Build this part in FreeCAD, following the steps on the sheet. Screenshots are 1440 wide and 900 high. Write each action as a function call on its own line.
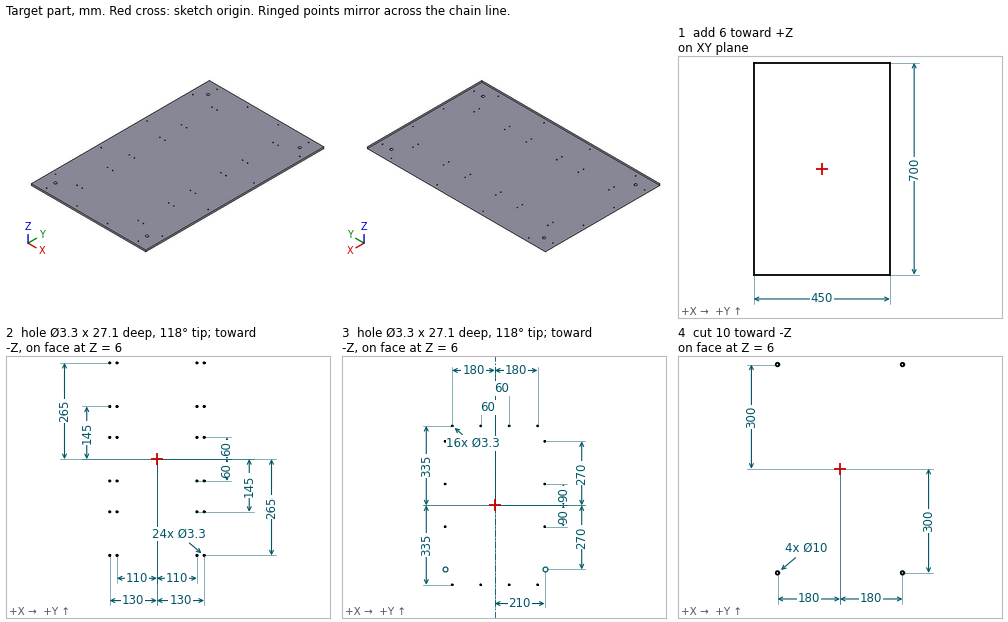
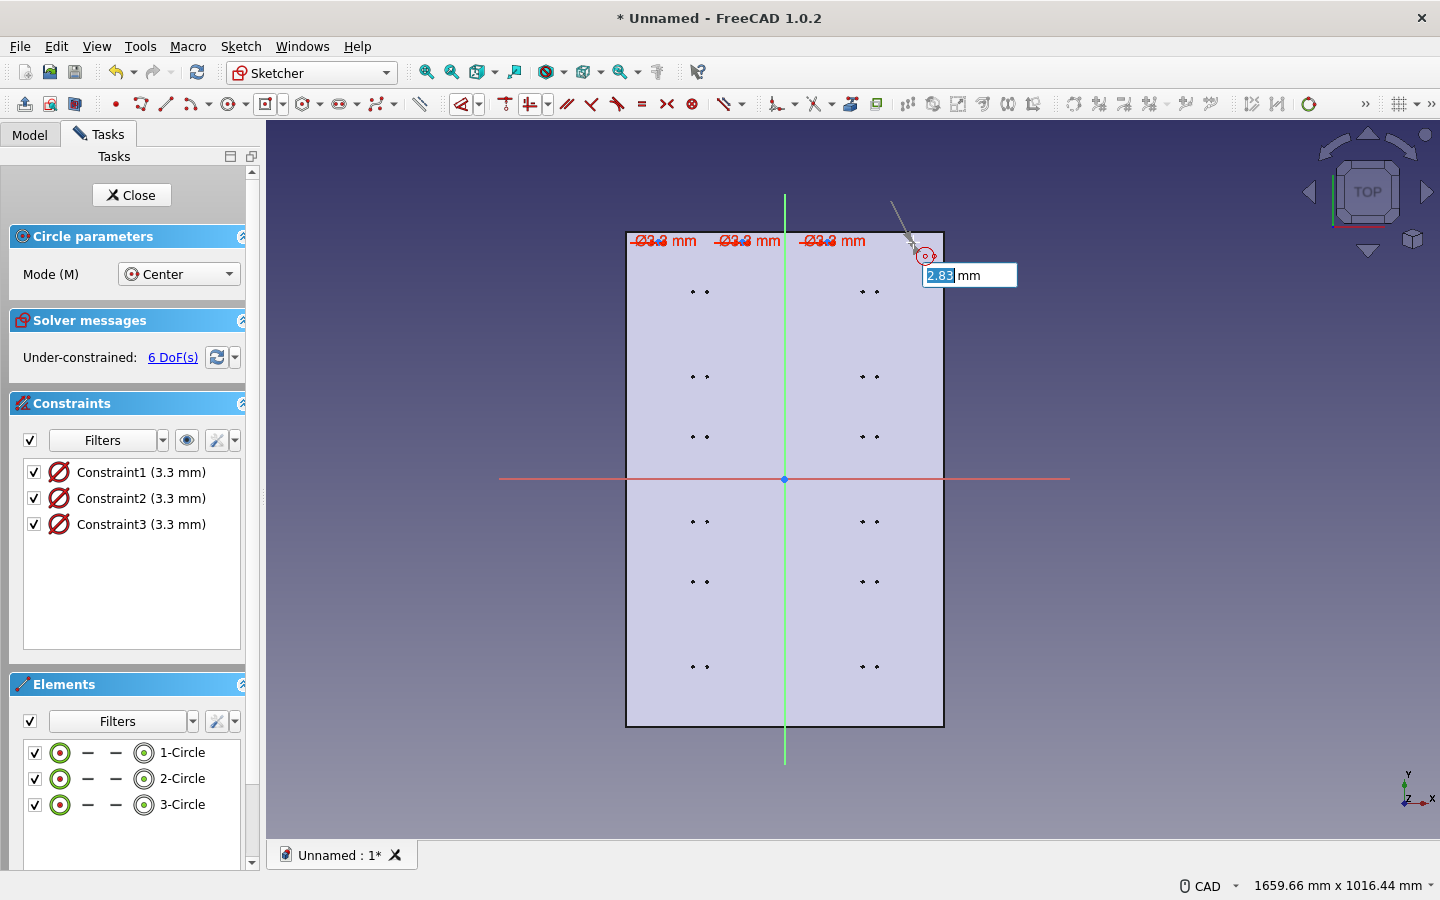
text(3.3)
key(Return)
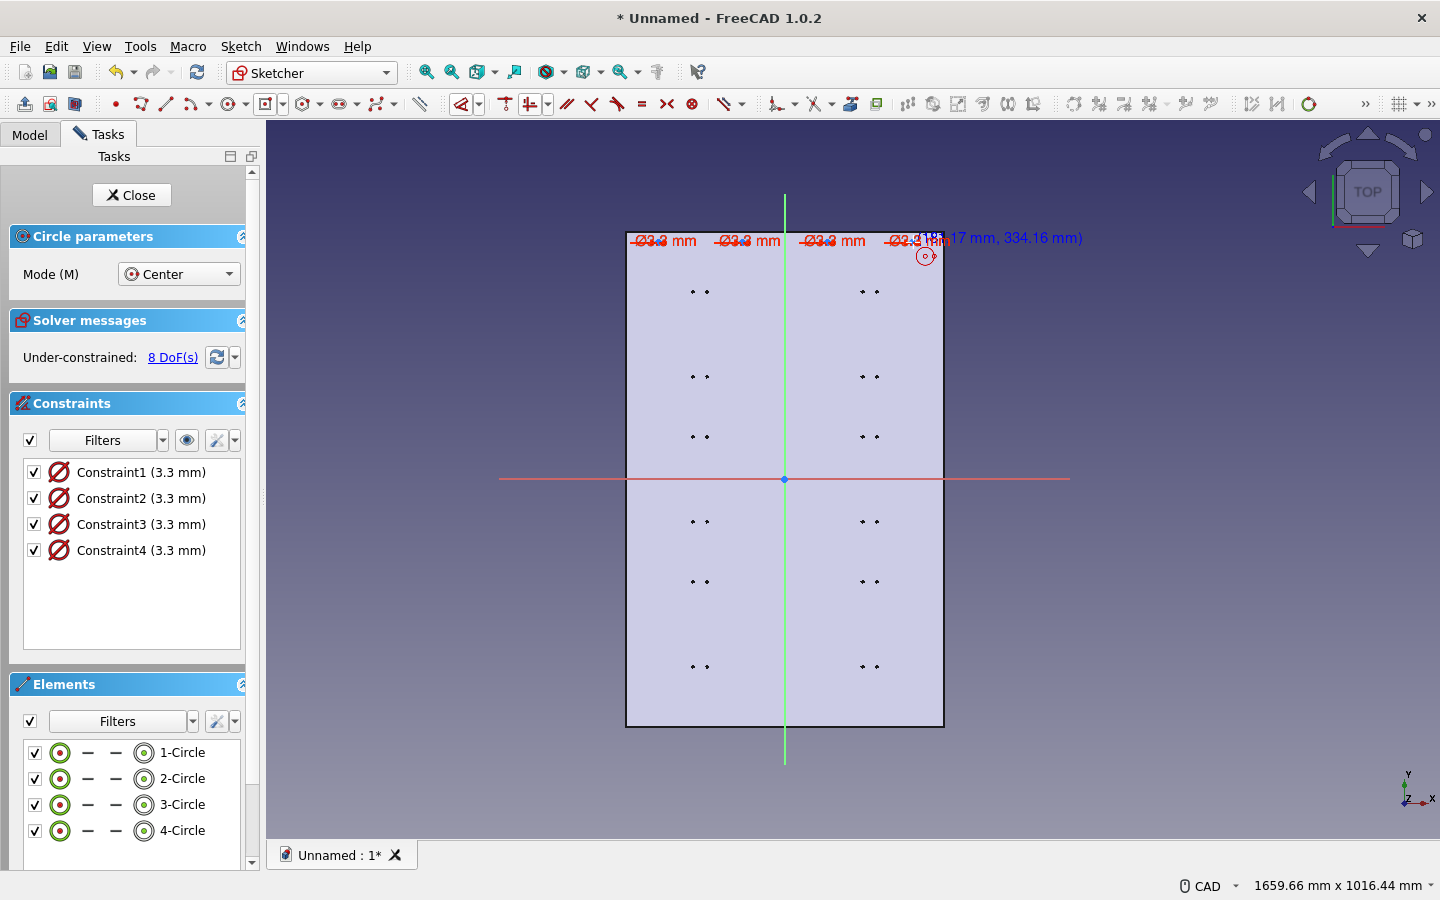
scroll(658, 716, up, 15)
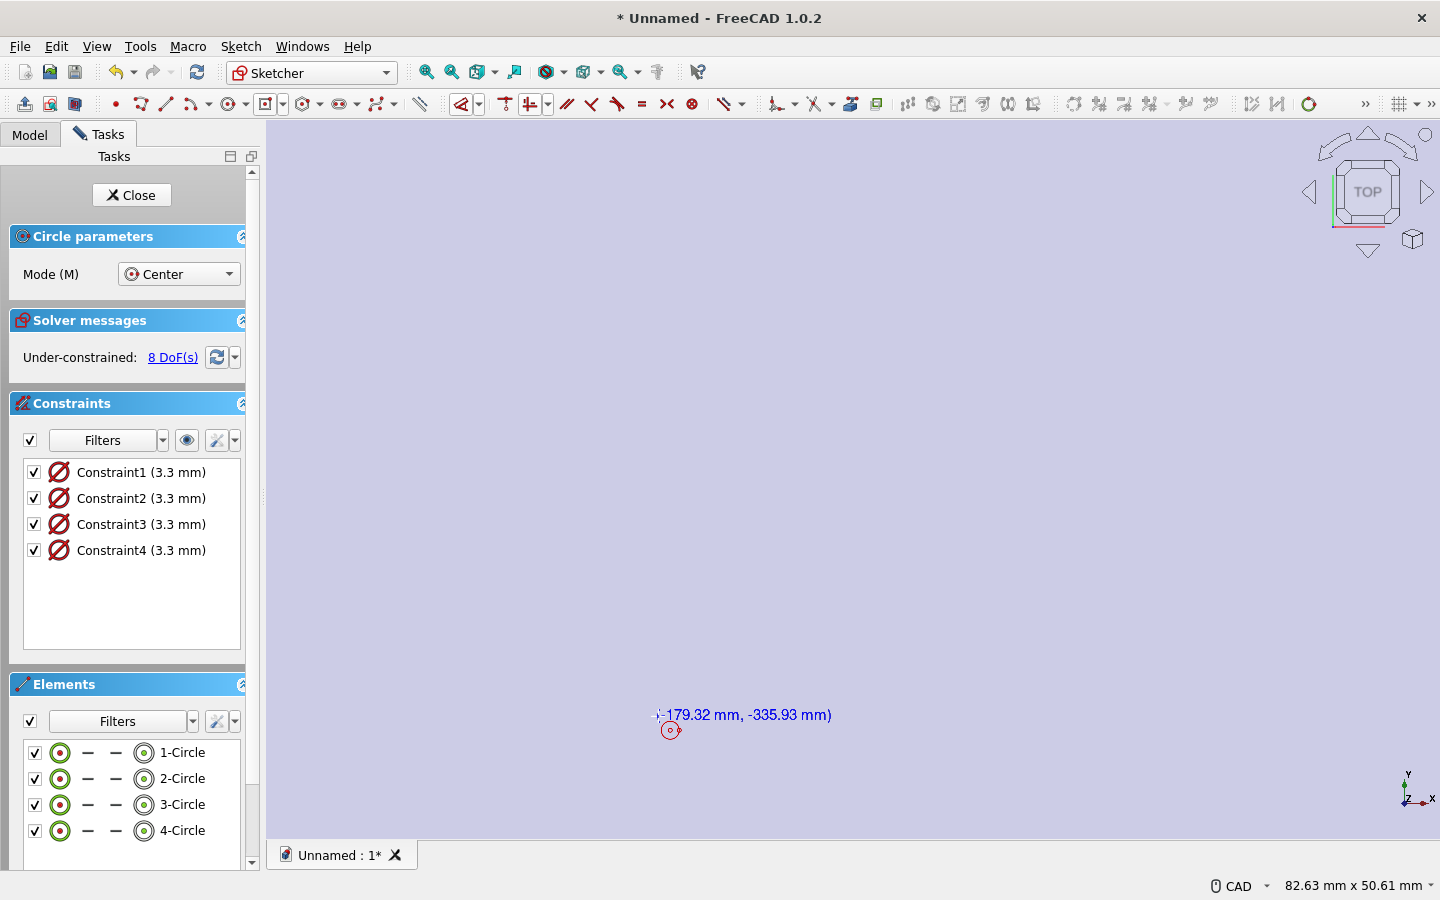
scroll(658, 717, down, 15)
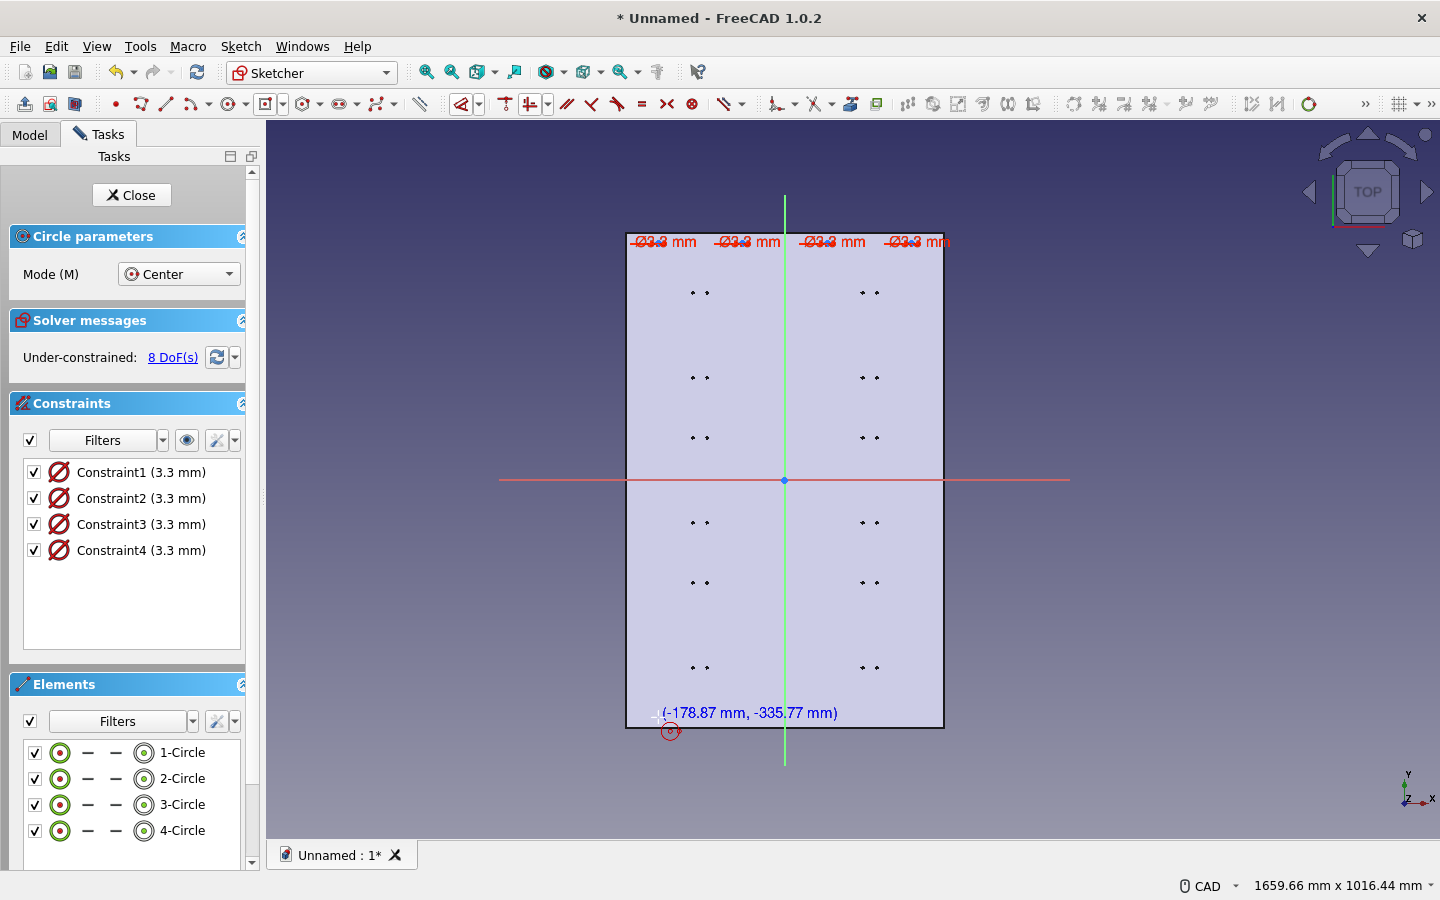
click(658, 717)
move(658, 716)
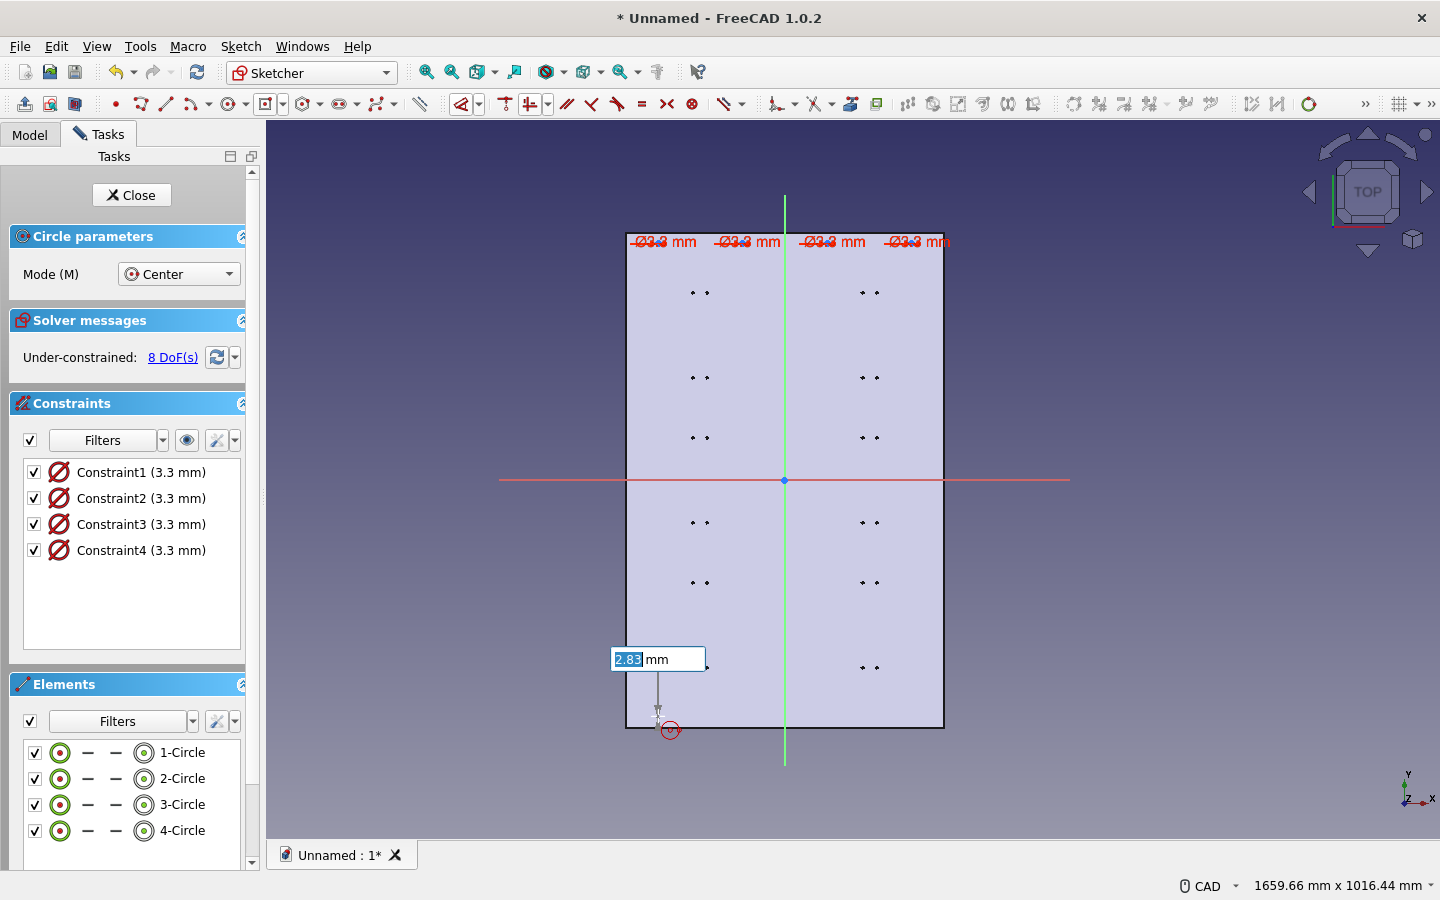
text(3.3)
key(Return)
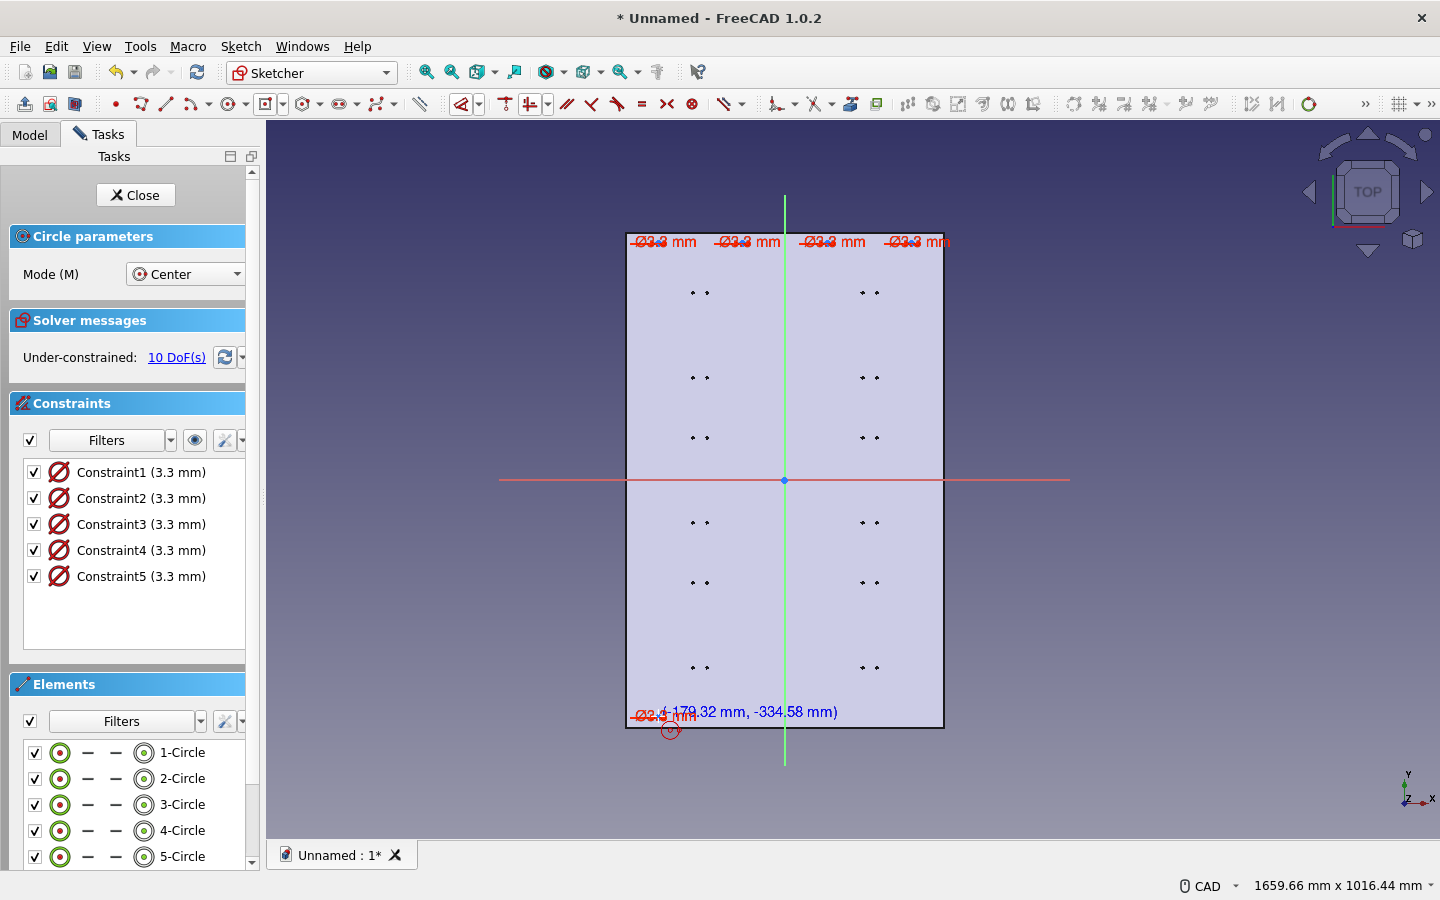
scroll(742, 717, up, 15)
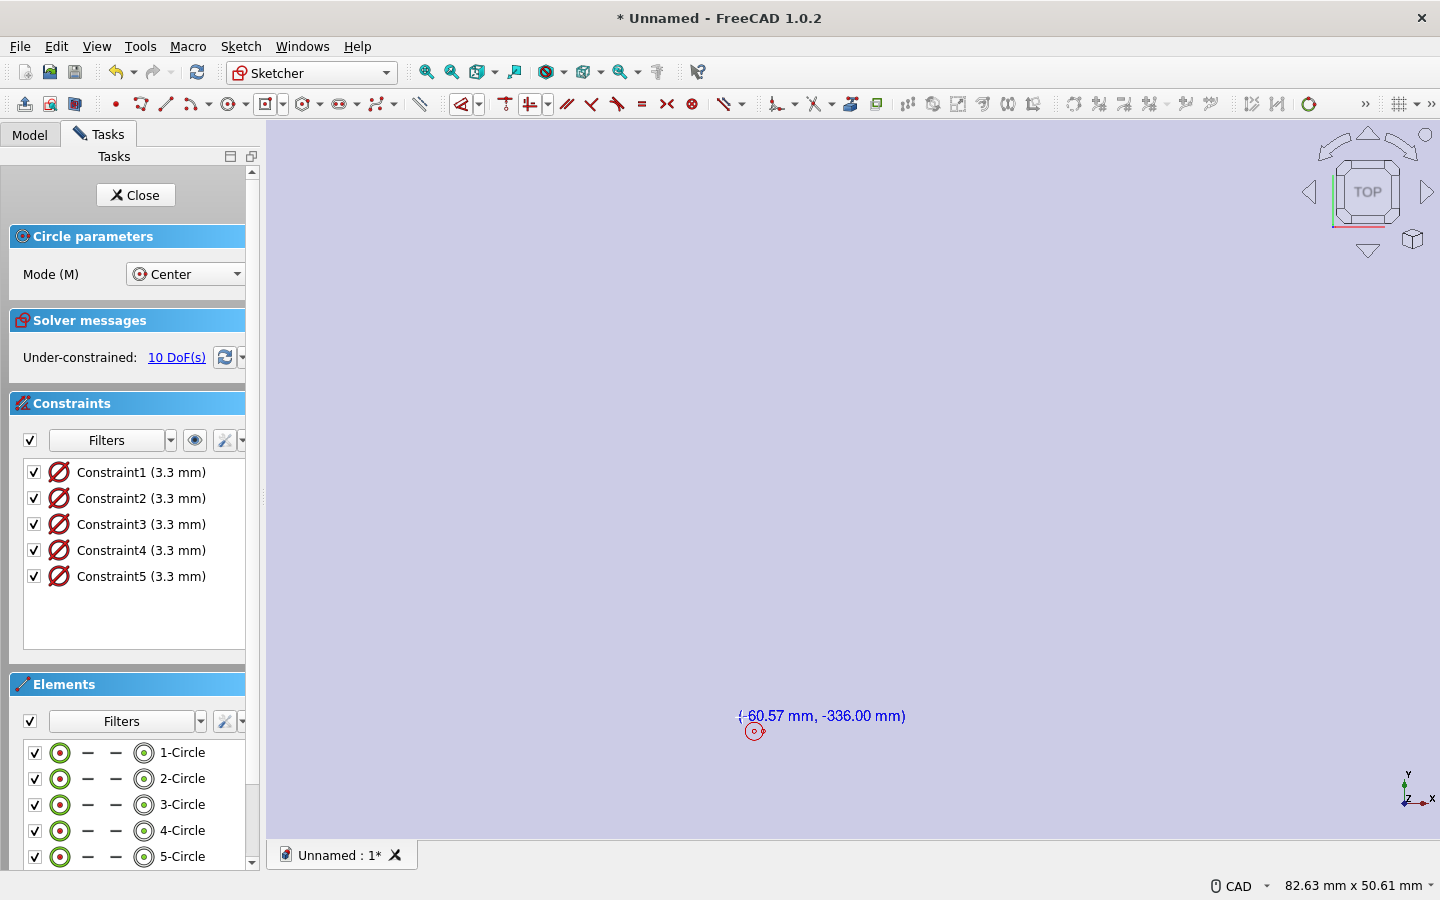
scroll(742, 717, down, 15)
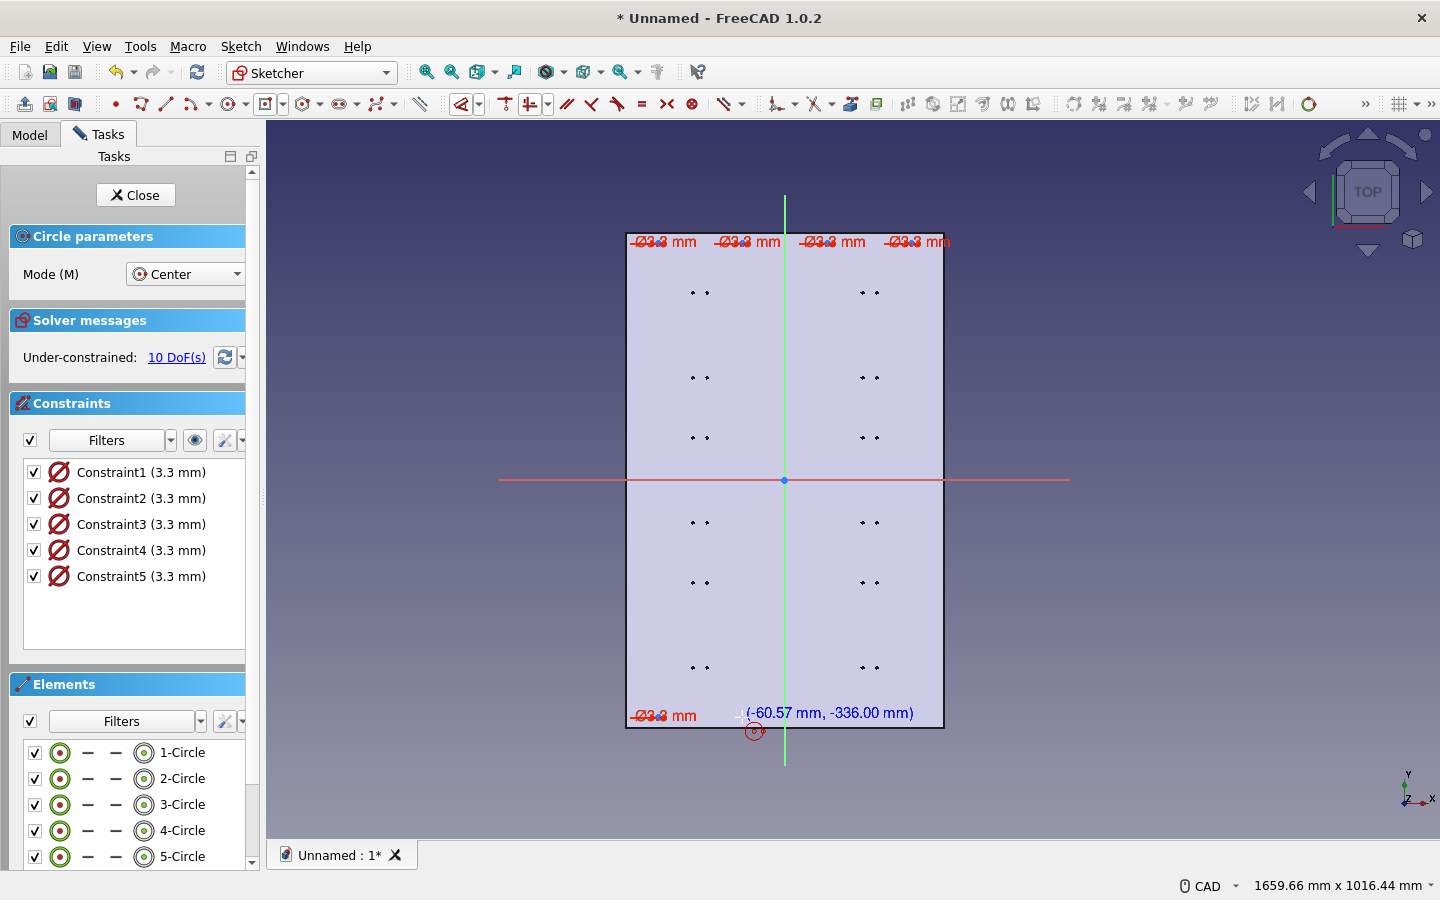
click(742, 717)
move(743, 716)